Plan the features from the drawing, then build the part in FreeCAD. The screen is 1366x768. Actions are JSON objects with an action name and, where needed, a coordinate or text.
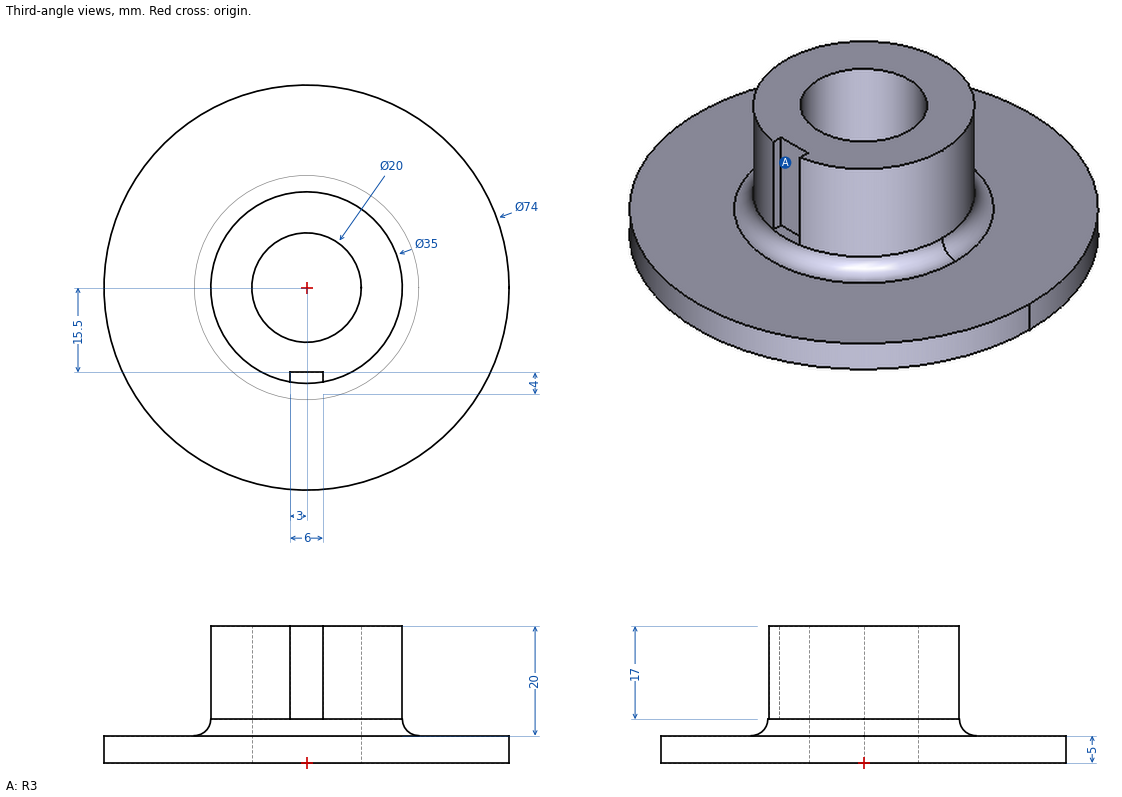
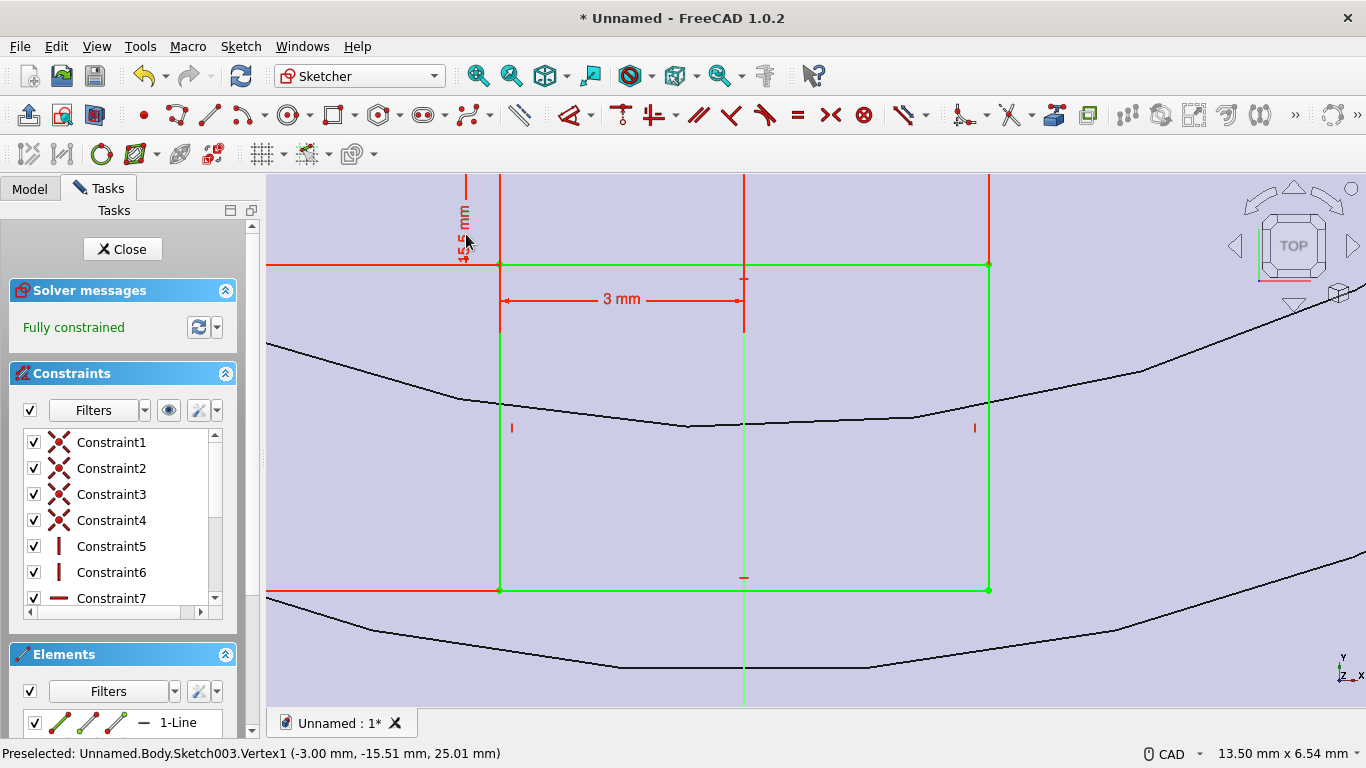
{"action": "left_click", "coordinate": [123, 249]}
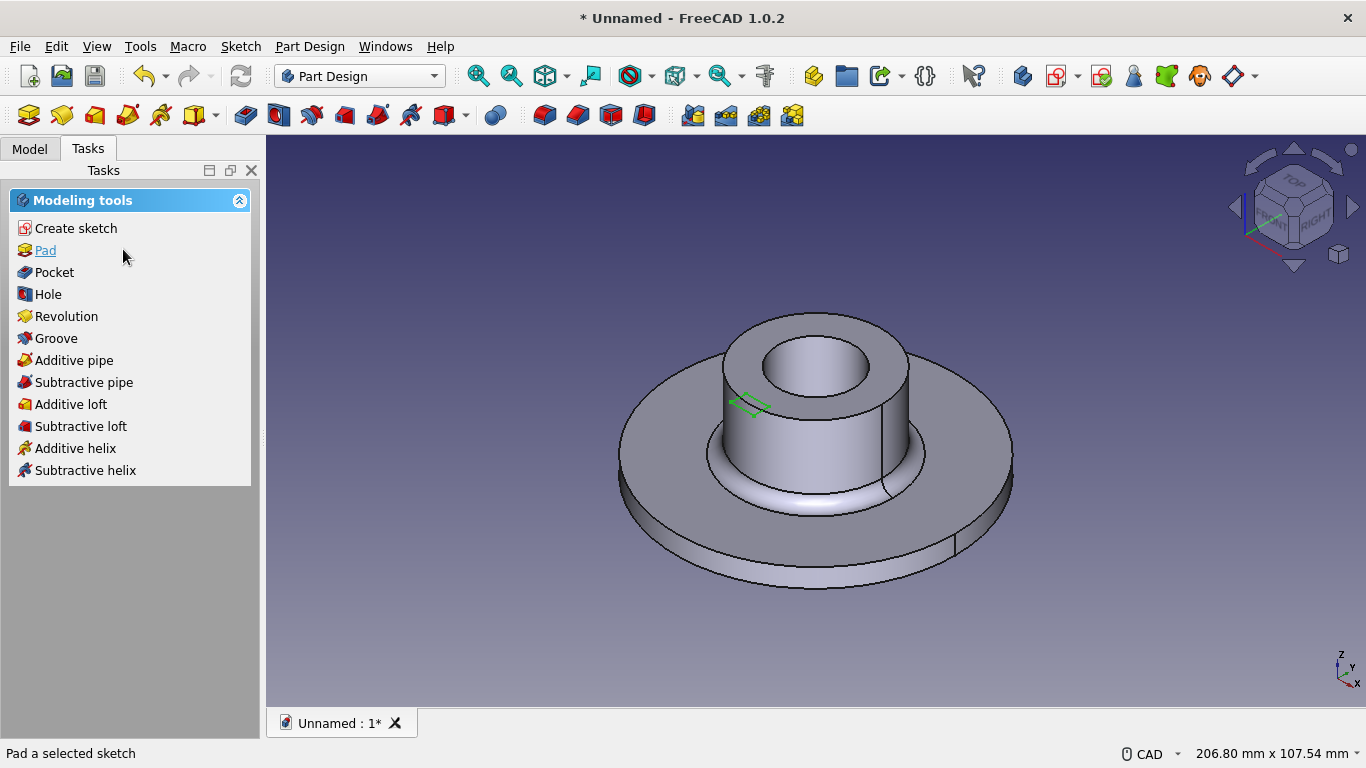
{"action": "left_click", "coordinate": [246, 116]}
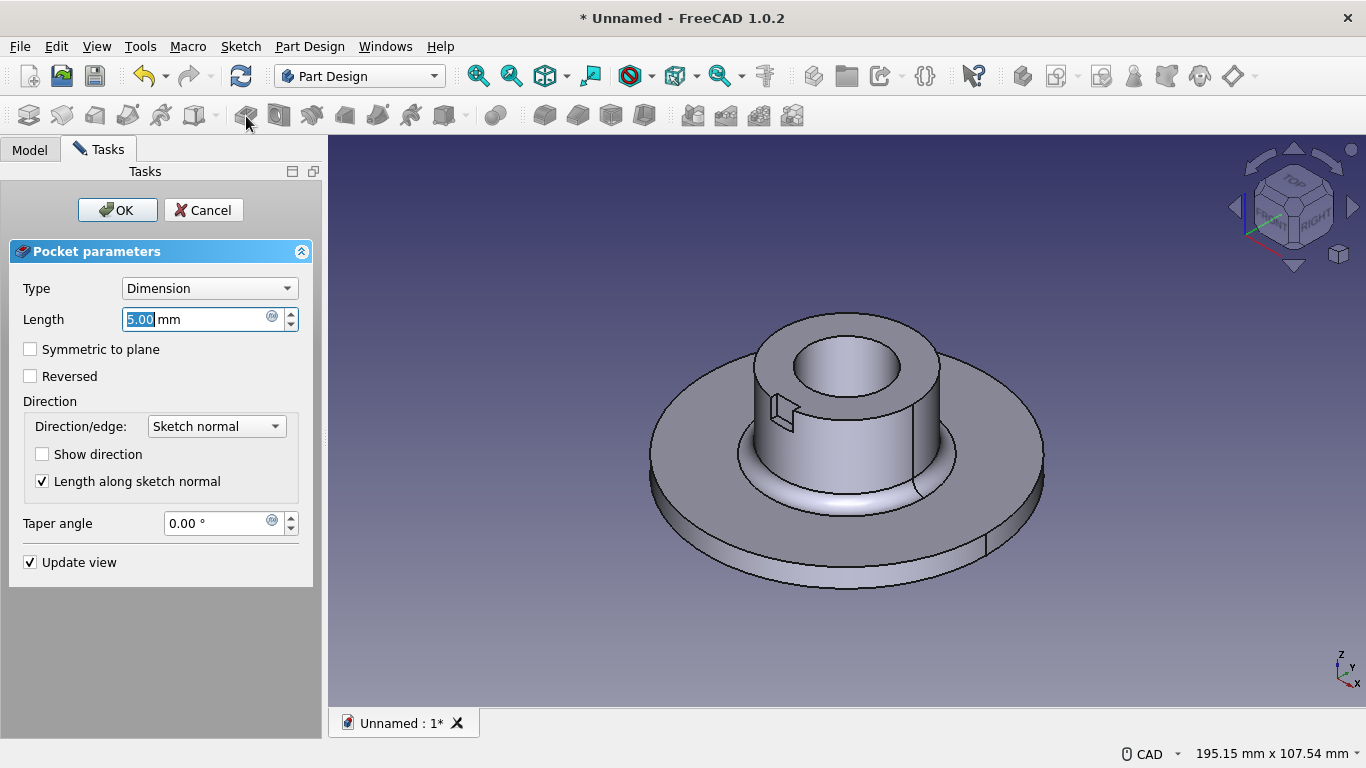
{"action": "type", "text": "17"}
{"action": "key", "text": "Tab"}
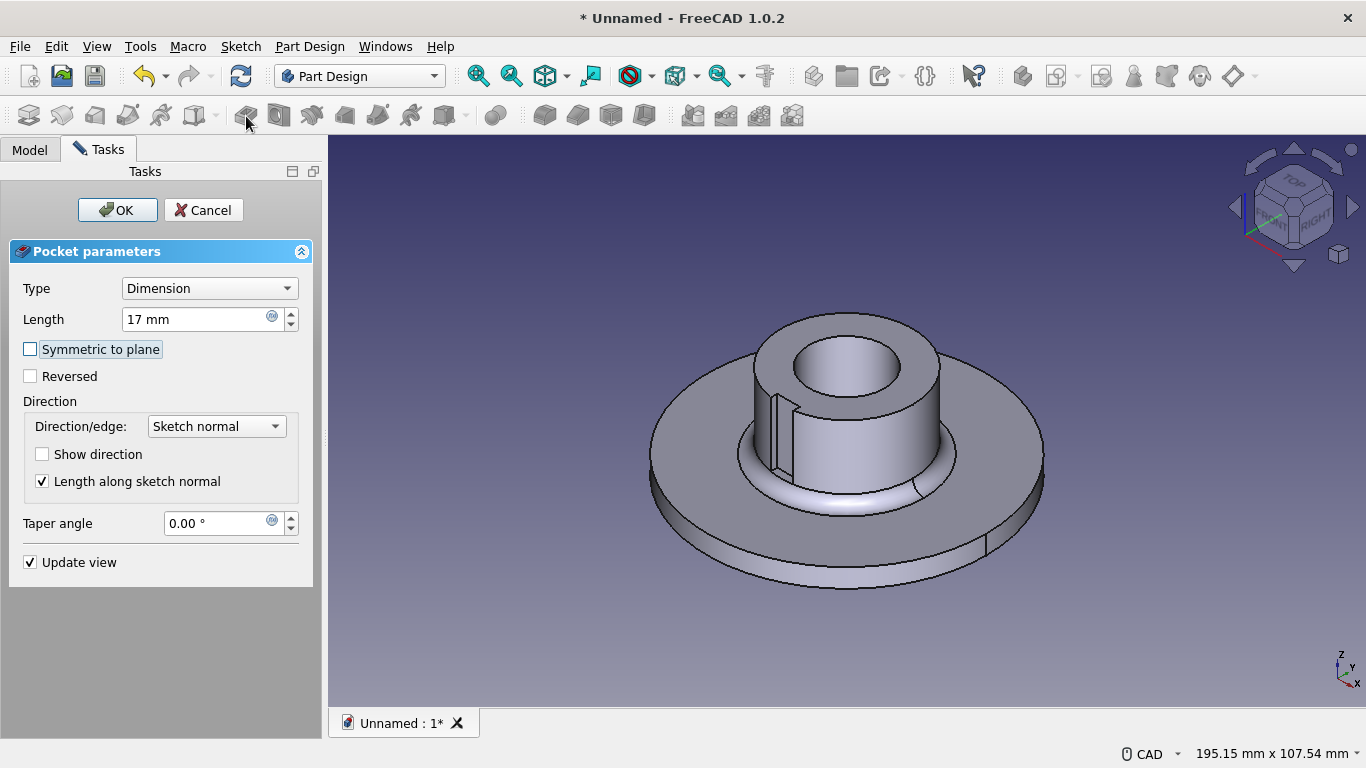
{"action": "left_click", "coordinate": [118, 210]}